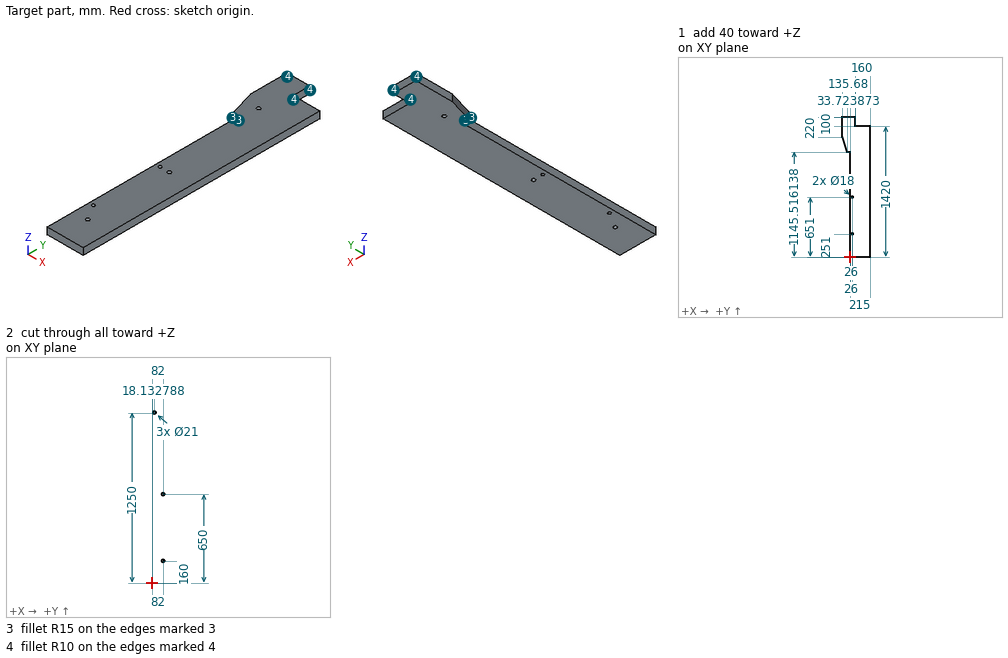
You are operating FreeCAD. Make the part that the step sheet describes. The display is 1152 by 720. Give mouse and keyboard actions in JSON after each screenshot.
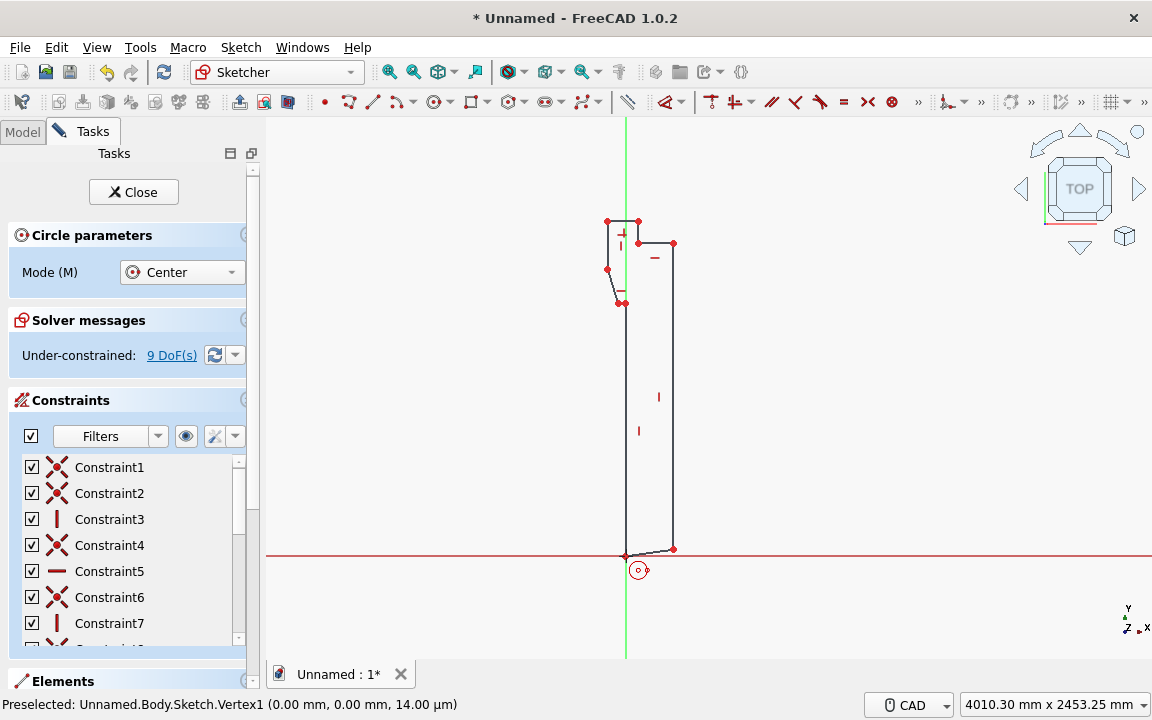
{"action": "scroll", "coordinate": [632, 501], "scroll_direction": "up", "scroll_amount": 13}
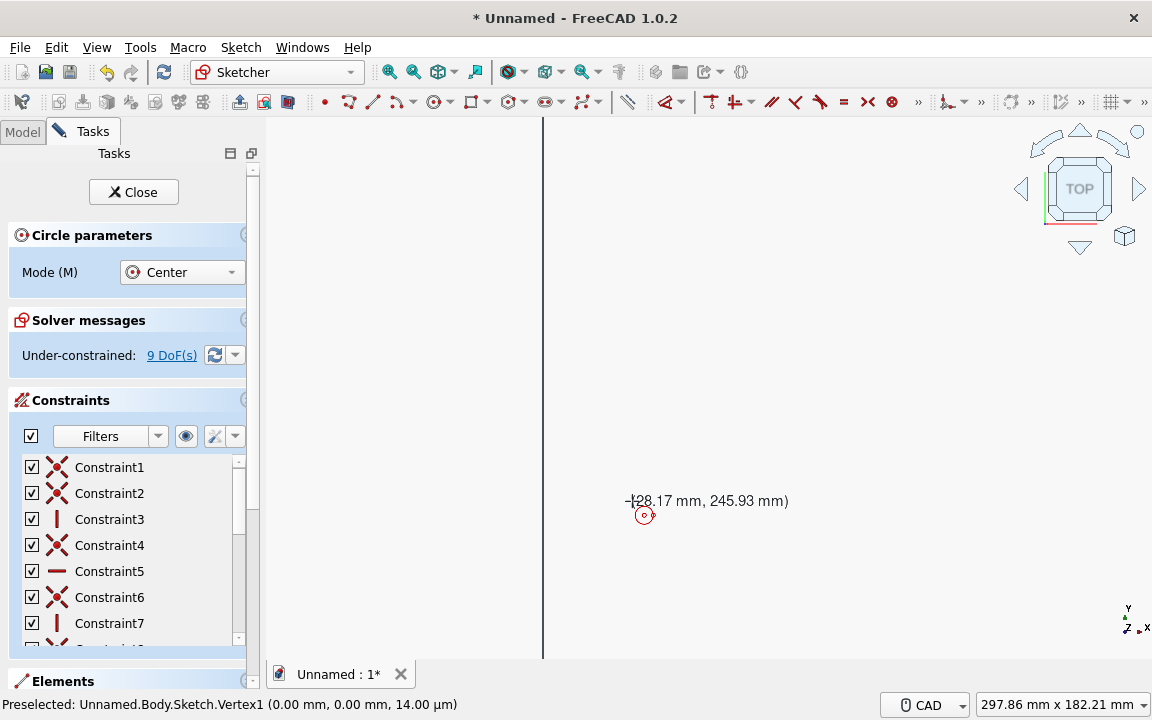
{"action": "scroll", "coordinate": [632, 501], "scroll_direction": "down", "scroll_amount": 13}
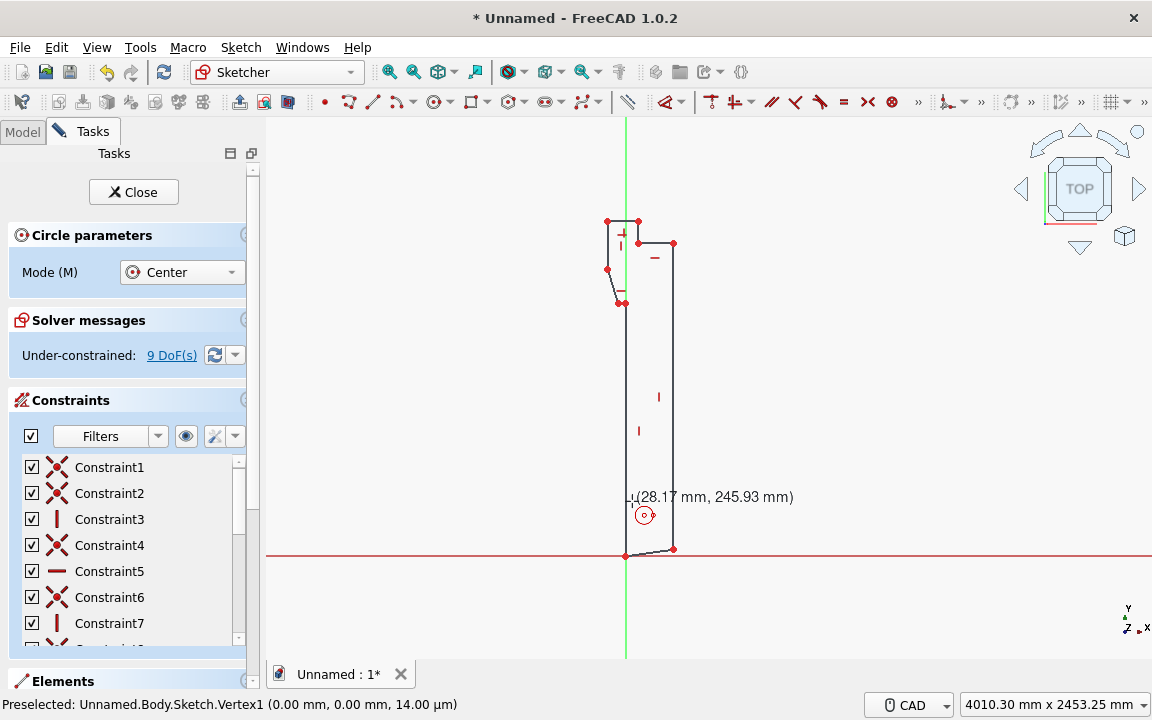
{"action": "scroll", "coordinate": [632, 501], "scroll_direction": "up", "scroll_amount": 6}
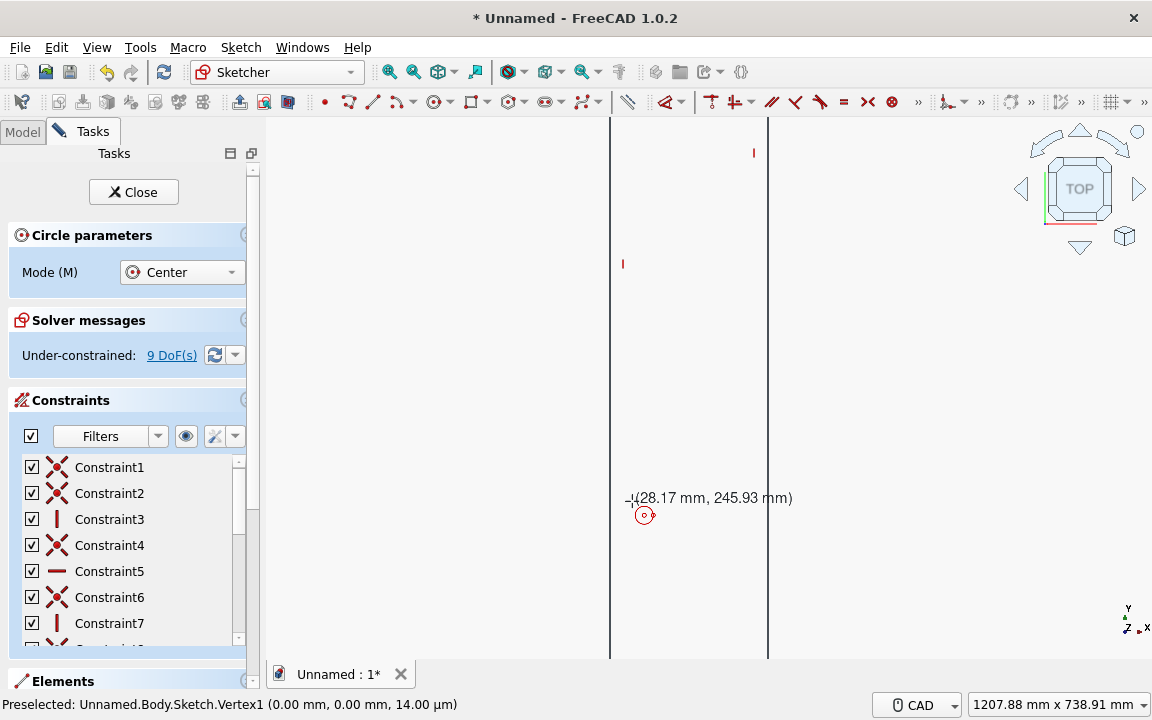
{"action": "left_click", "coordinate": [629, 499]}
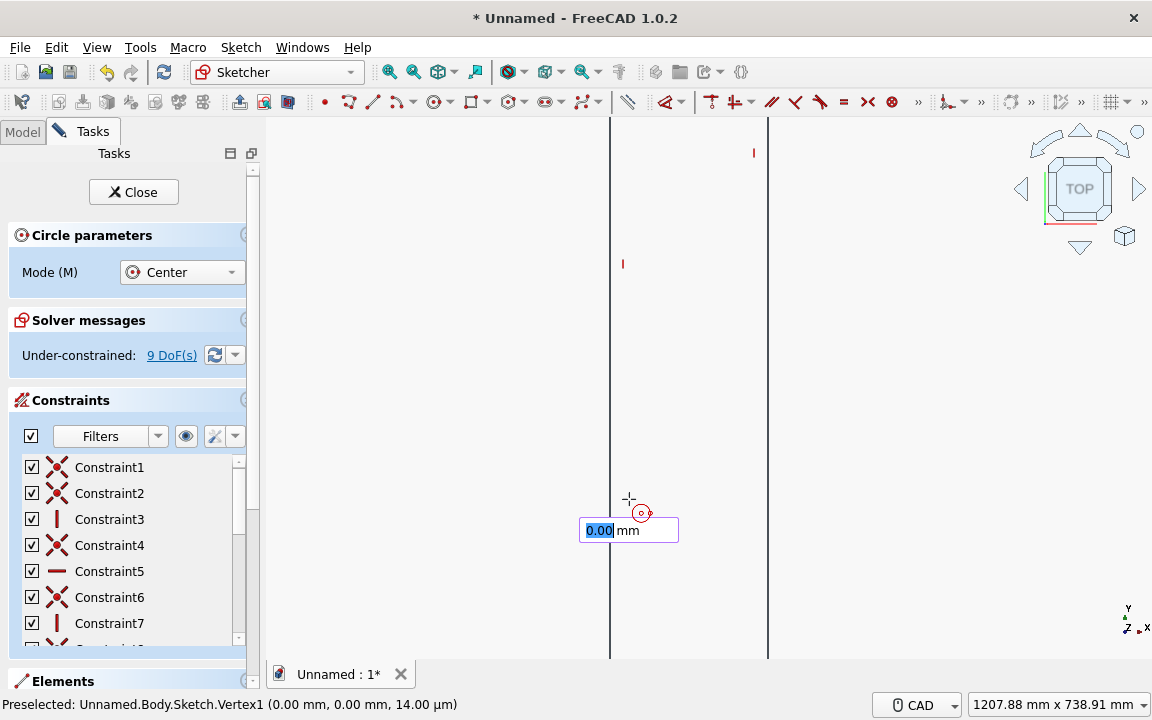
{"action": "scroll", "coordinate": [634, 494], "scroll_direction": "up", "scroll_amount": 5}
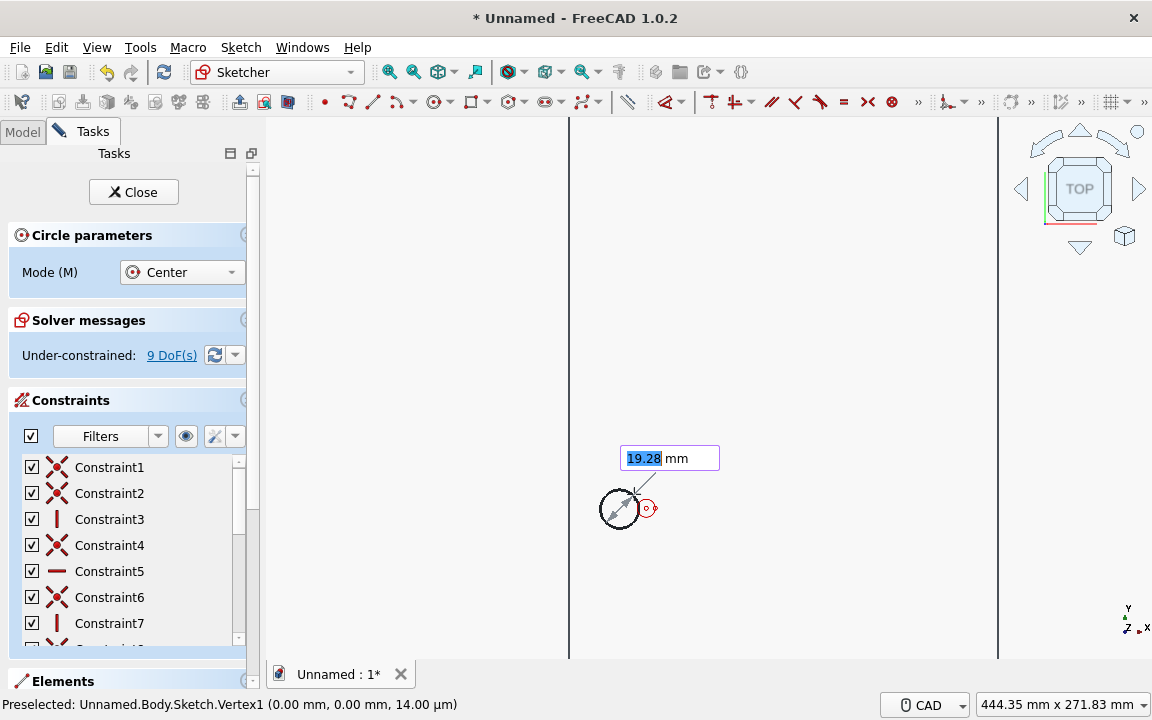
{"action": "left_click", "coordinate": [634, 494]}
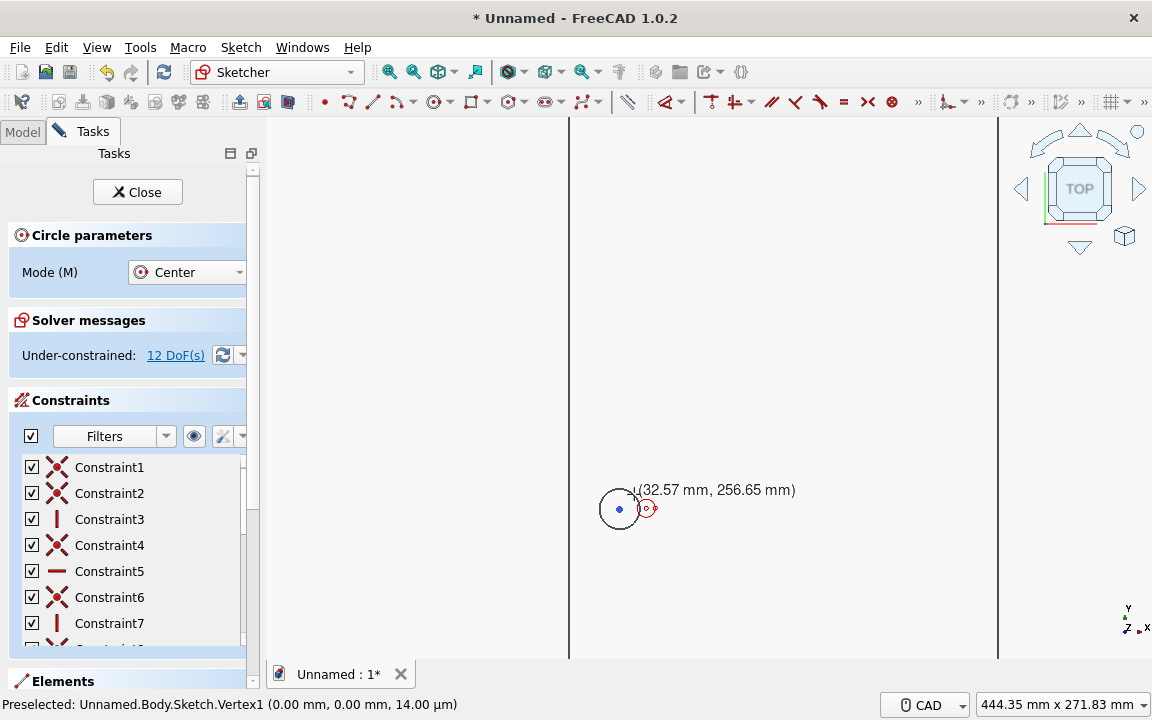
{"action": "scroll", "coordinate": [633, 500], "scroll_direction": "down", "scroll_amount": 11}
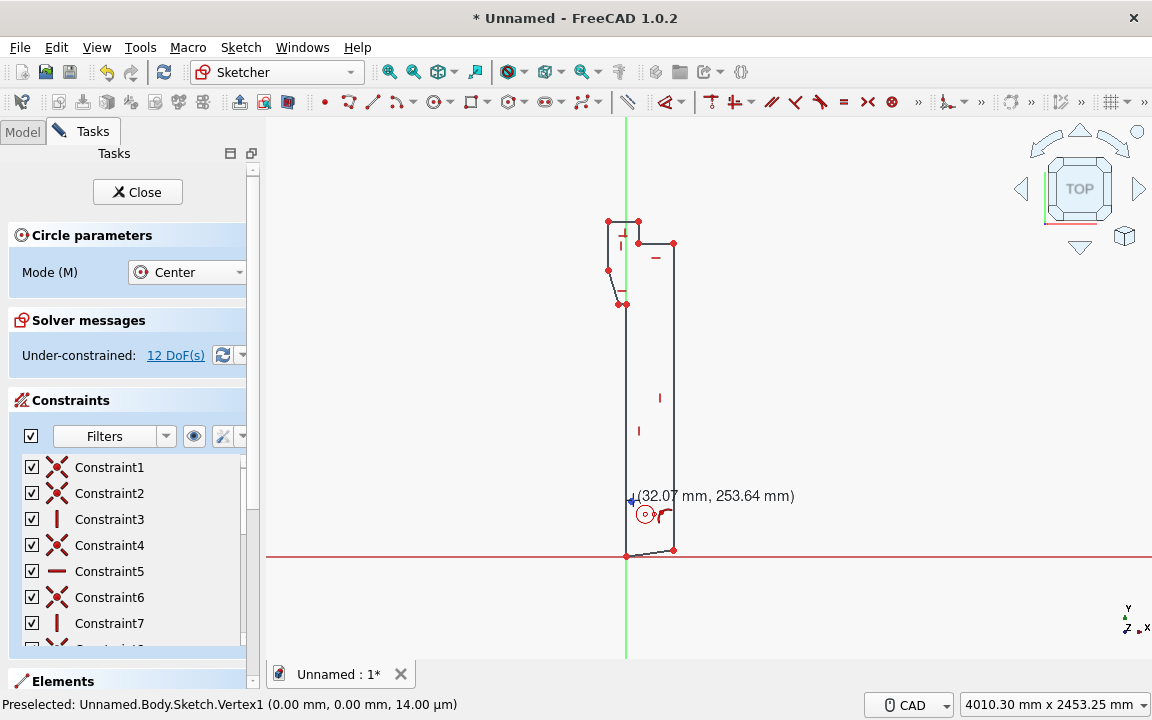
{"action": "scroll", "coordinate": [632, 413], "scroll_direction": "up", "scroll_amount": 13}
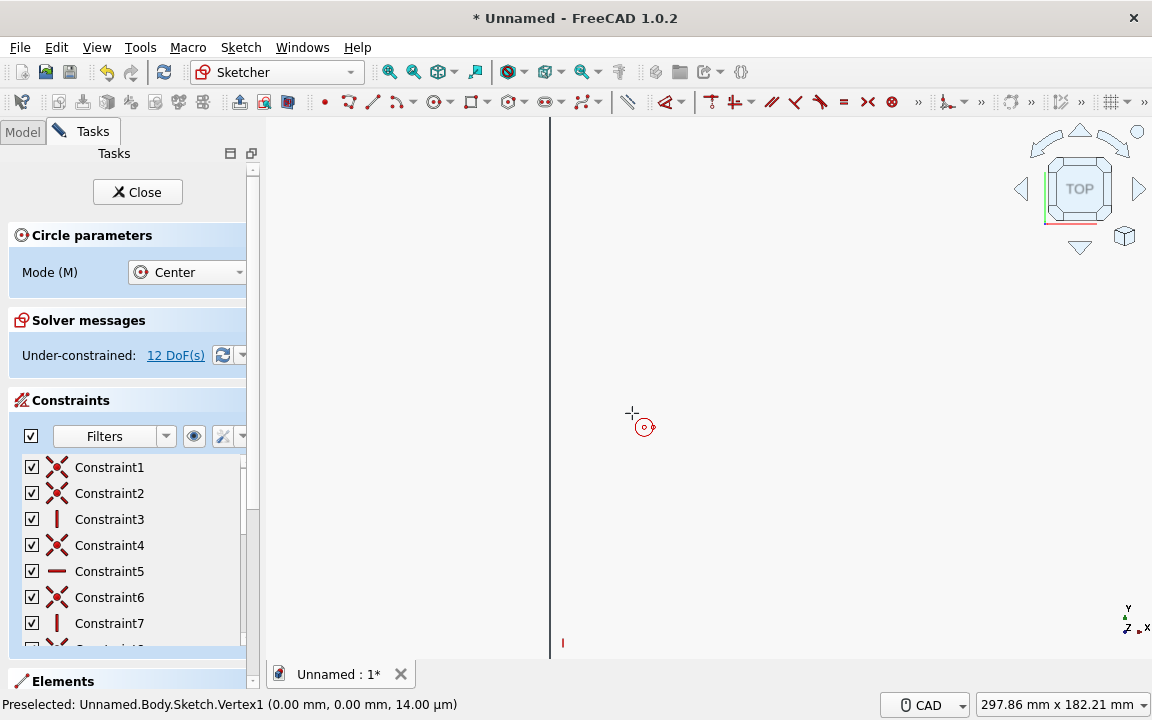
{"action": "scroll", "coordinate": [632, 413], "scroll_direction": "down", "scroll_amount": 13}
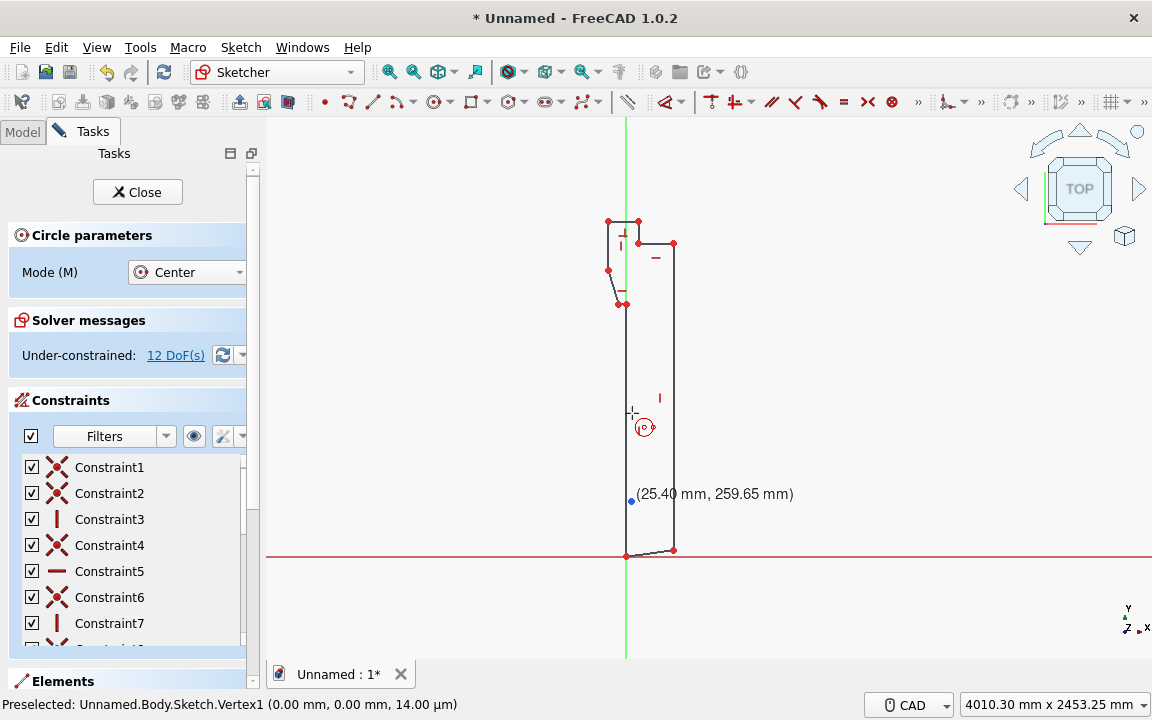
{"action": "scroll", "coordinate": [632, 413], "scroll_direction": "up", "scroll_amount": 6}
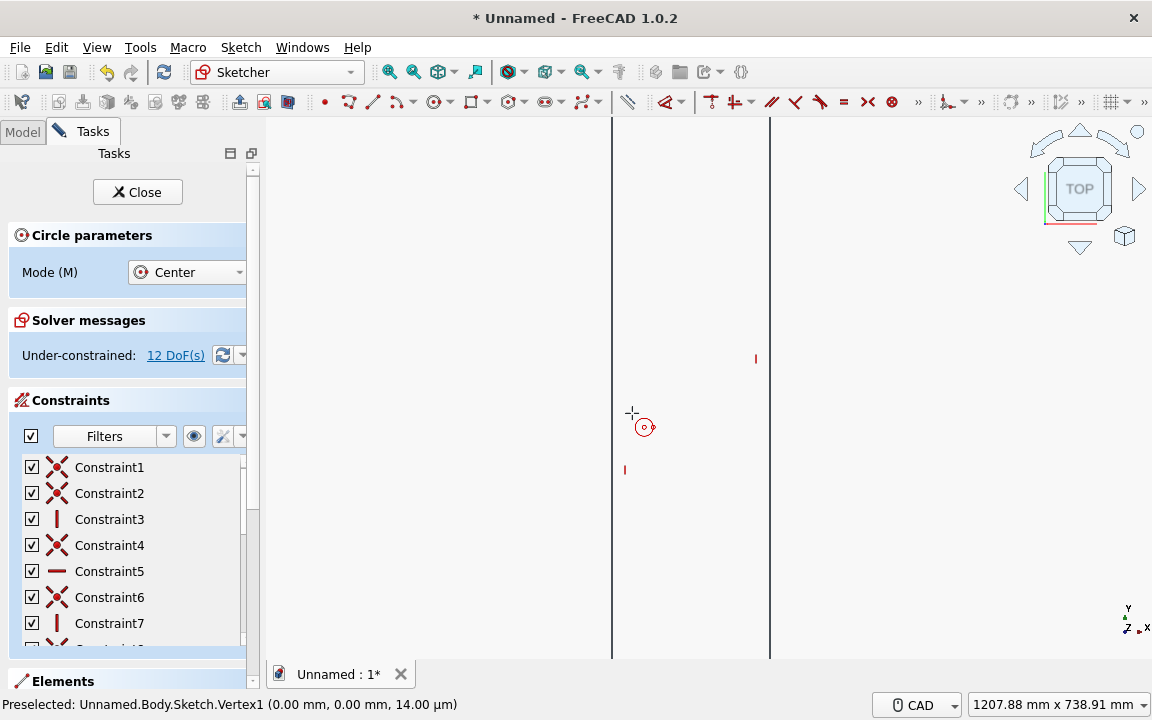
{"action": "left_click", "coordinate": [631, 412]}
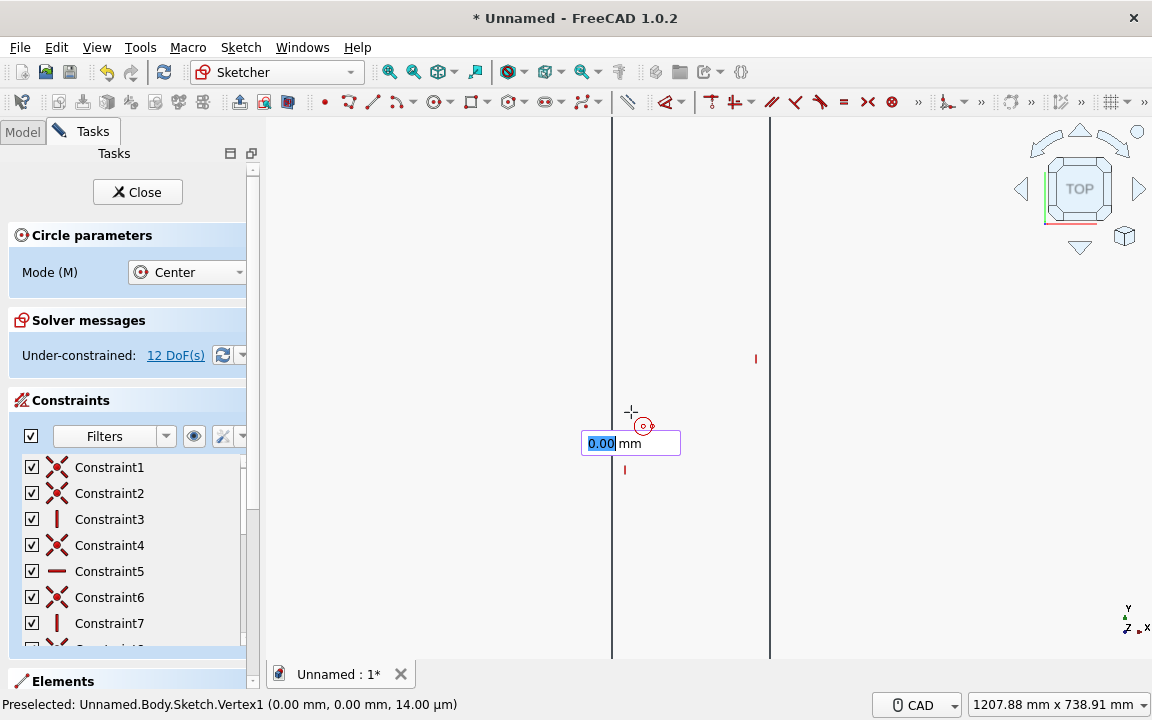
{"action": "scroll", "coordinate": [636, 407], "scroll_direction": "up", "scroll_amount": 5}